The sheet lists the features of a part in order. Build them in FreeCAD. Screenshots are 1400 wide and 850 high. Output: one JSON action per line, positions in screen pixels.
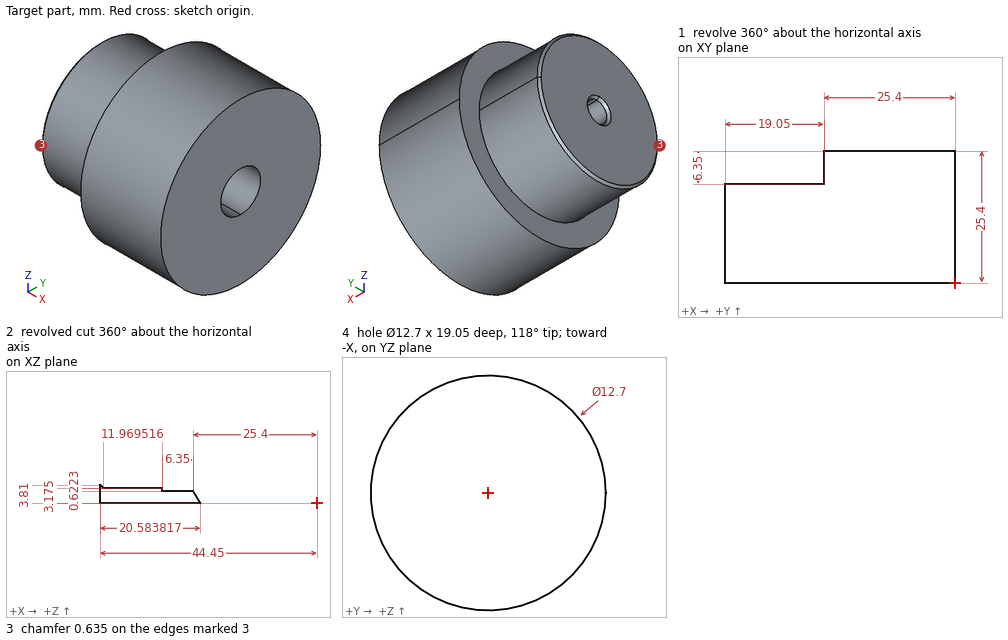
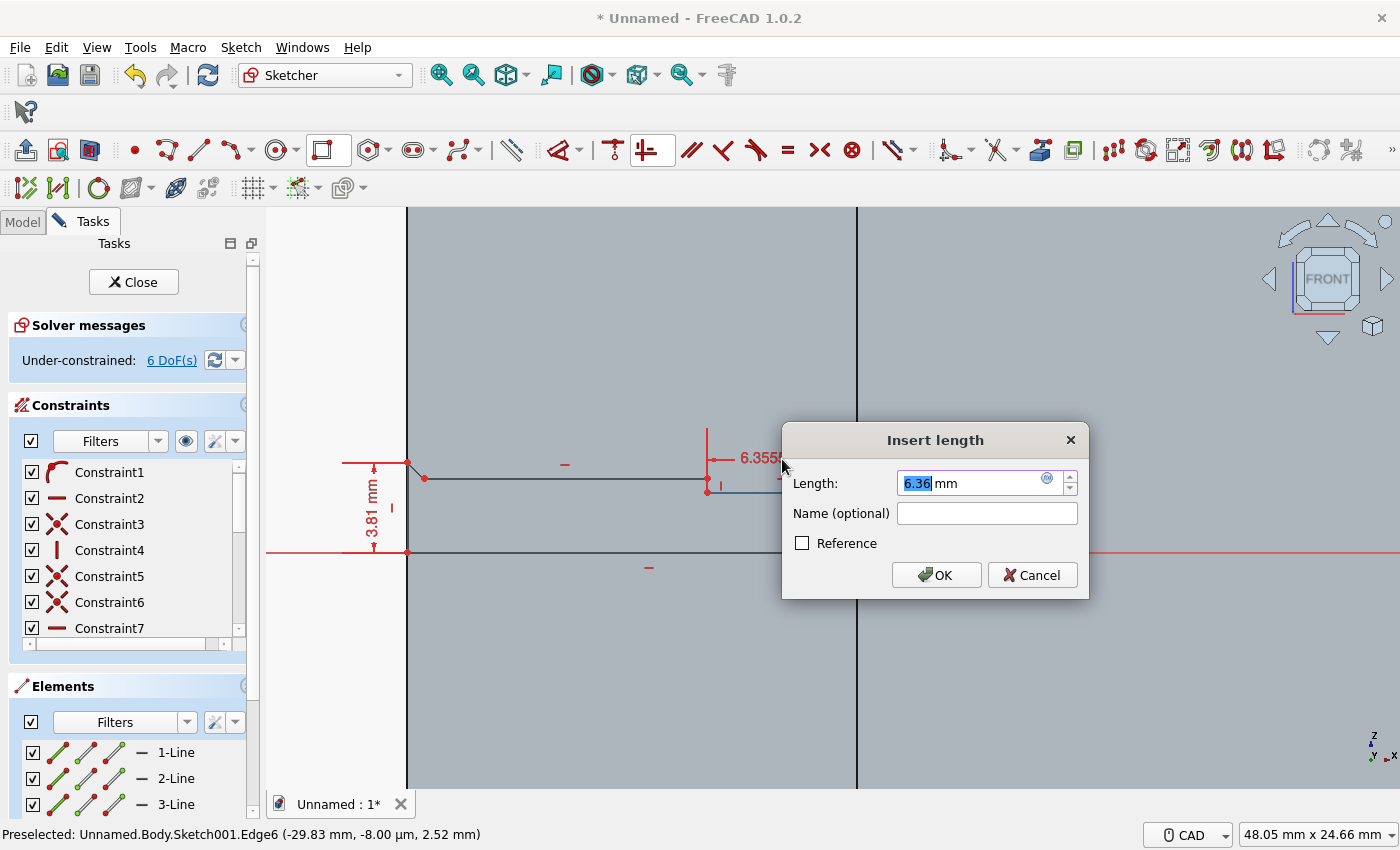
{"action": "type", "text": "6.35"}
{"action": "key", "text": "Return"}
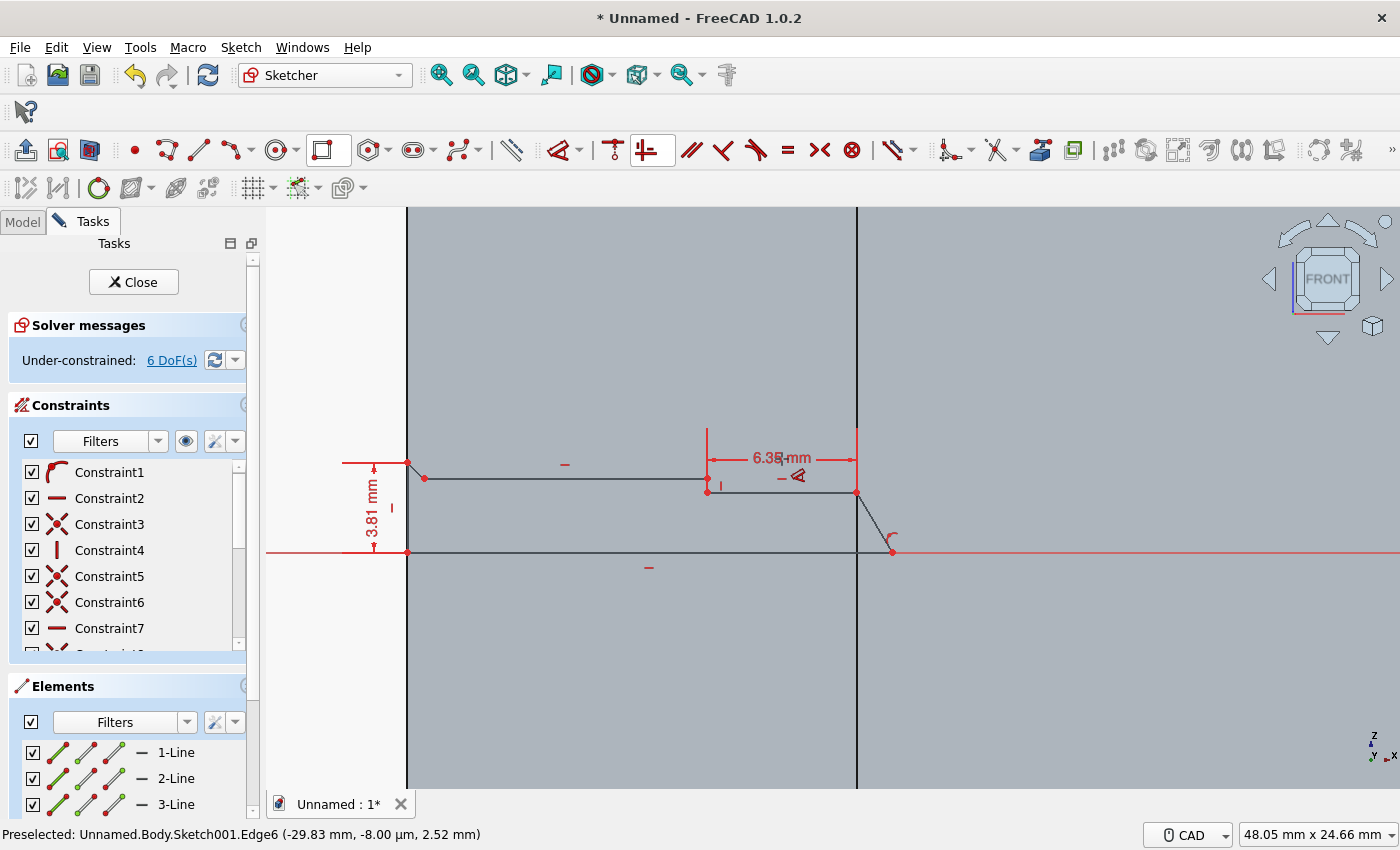
{"action": "left_click", "coordinate": [857, 493]}
{"action": "left_click", "coordinate": [1046, 587]}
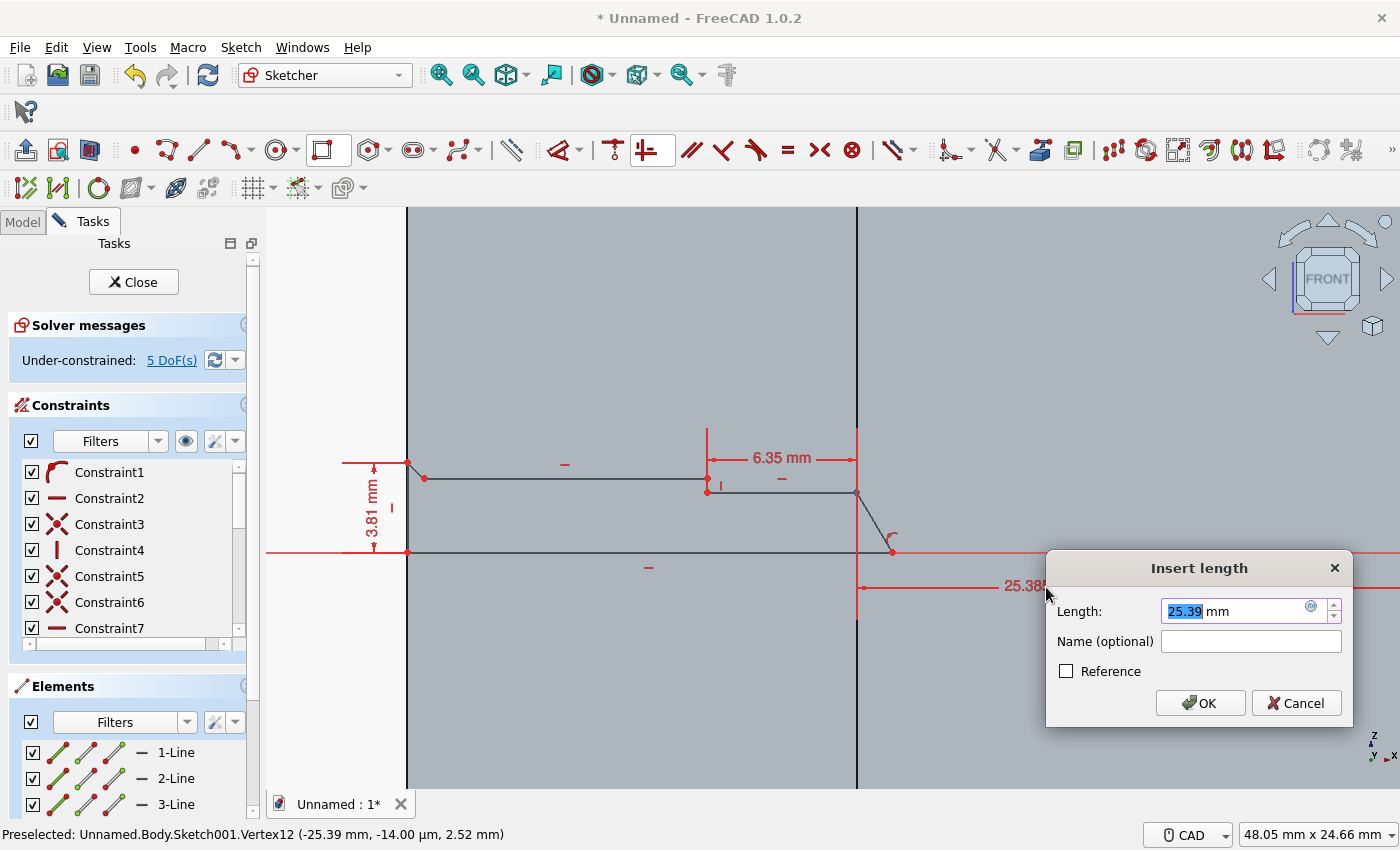
{"action": "type", "text": "25.4"}
{"action": "key", "text": "Return"}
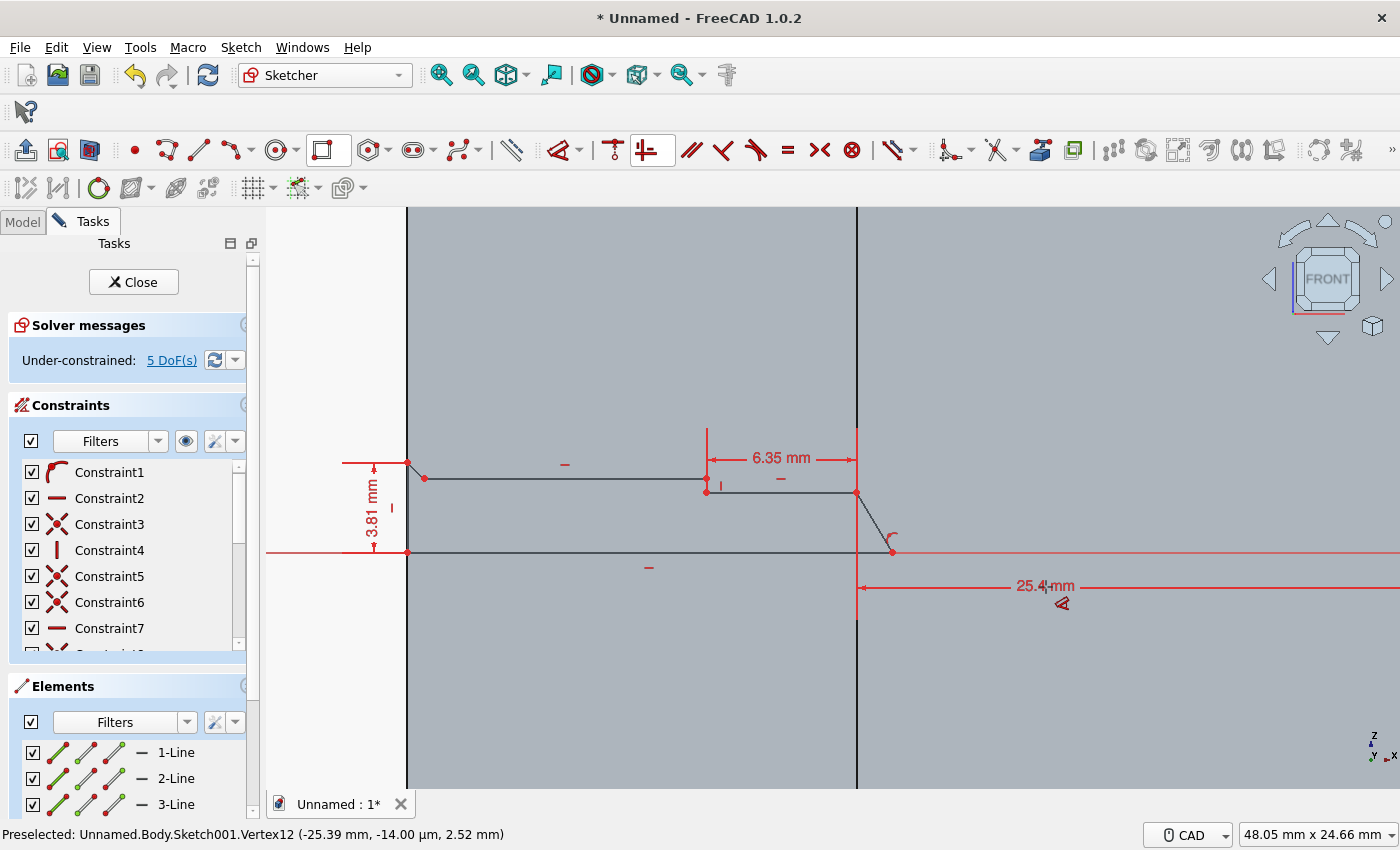
{"action": "scroll", "coordinate": [707, 486], "scroll_direction": "up", "scroll_amount": 5}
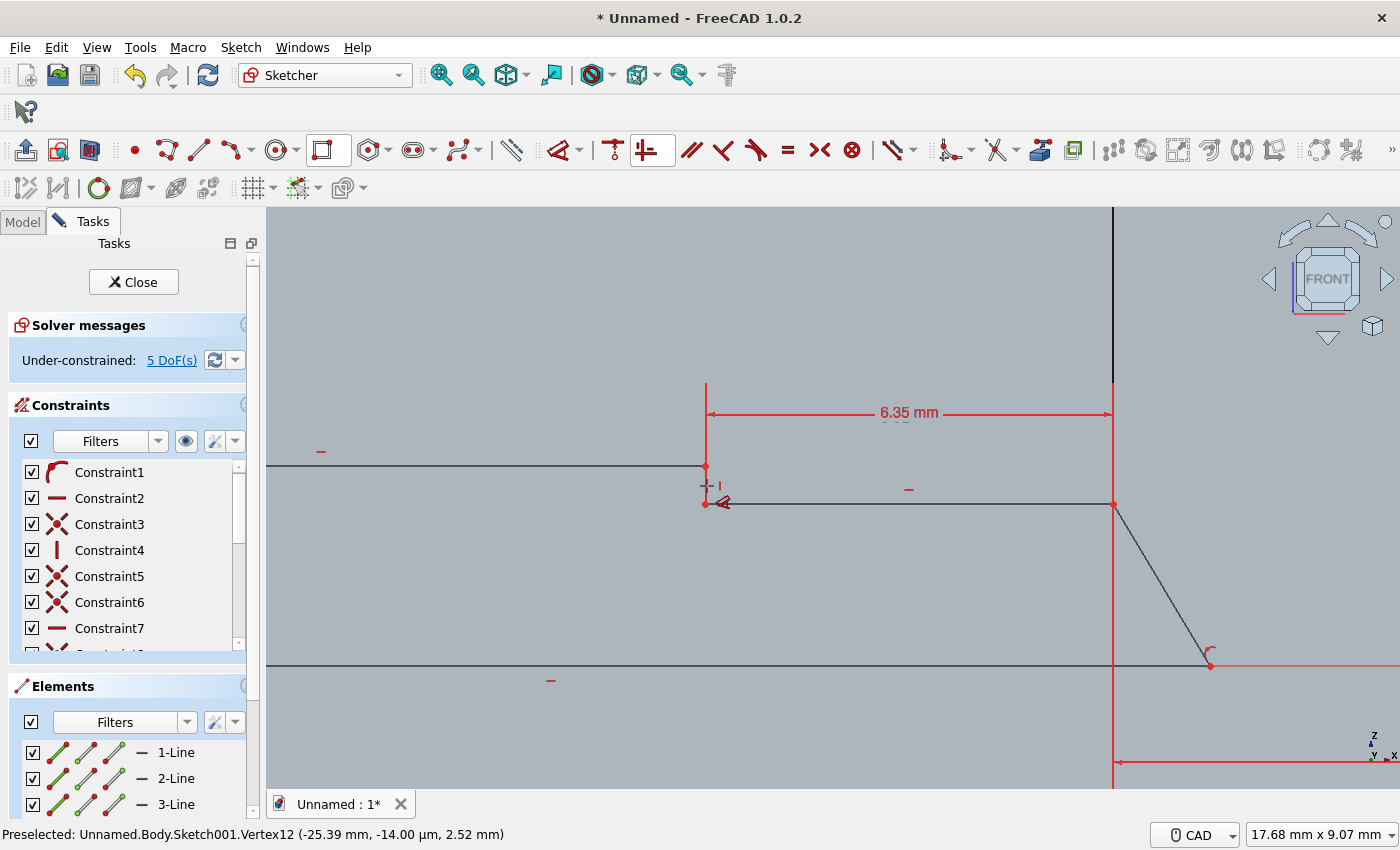
{"action": "left_click", "coordinate": [706, 485]}
{"action": "left_click", "coordinate": [672, 485]}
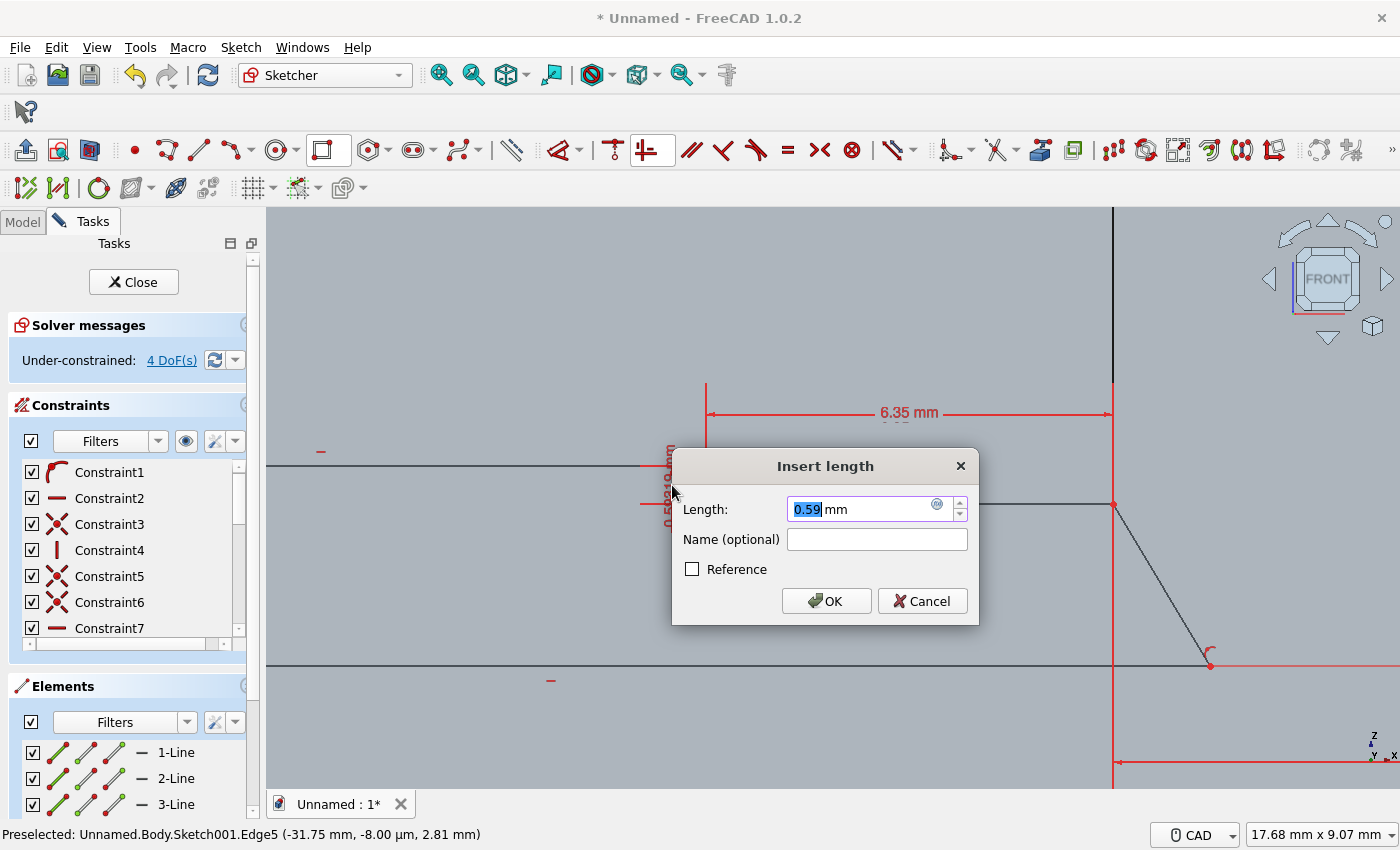
{"action": "type", "text": "0.6223"}
{"action": "key", "text": "Return"}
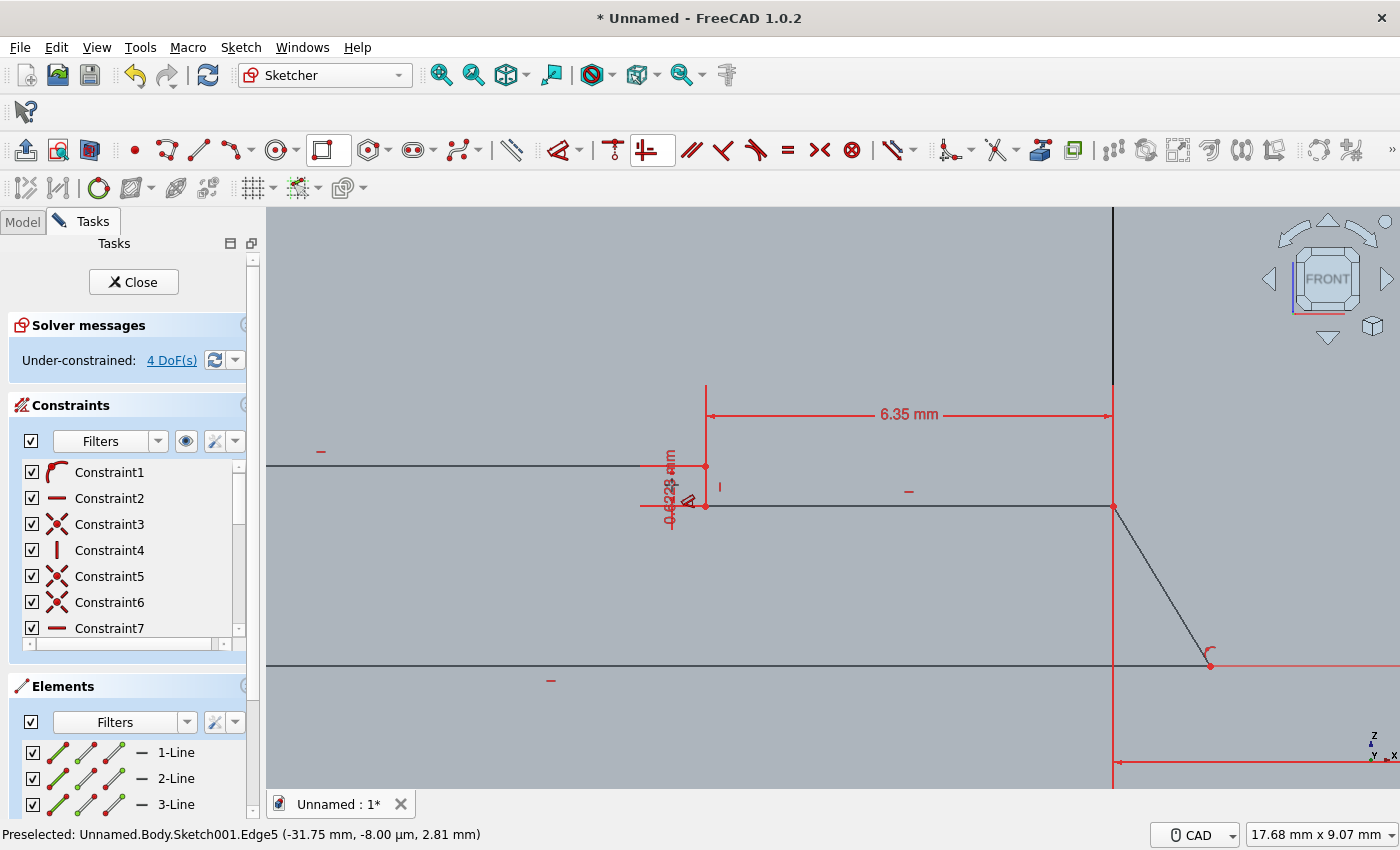
{"action": "scroll", "coordinate": [584, 483], "scroll_direction": "down", "scroll_amount": 7}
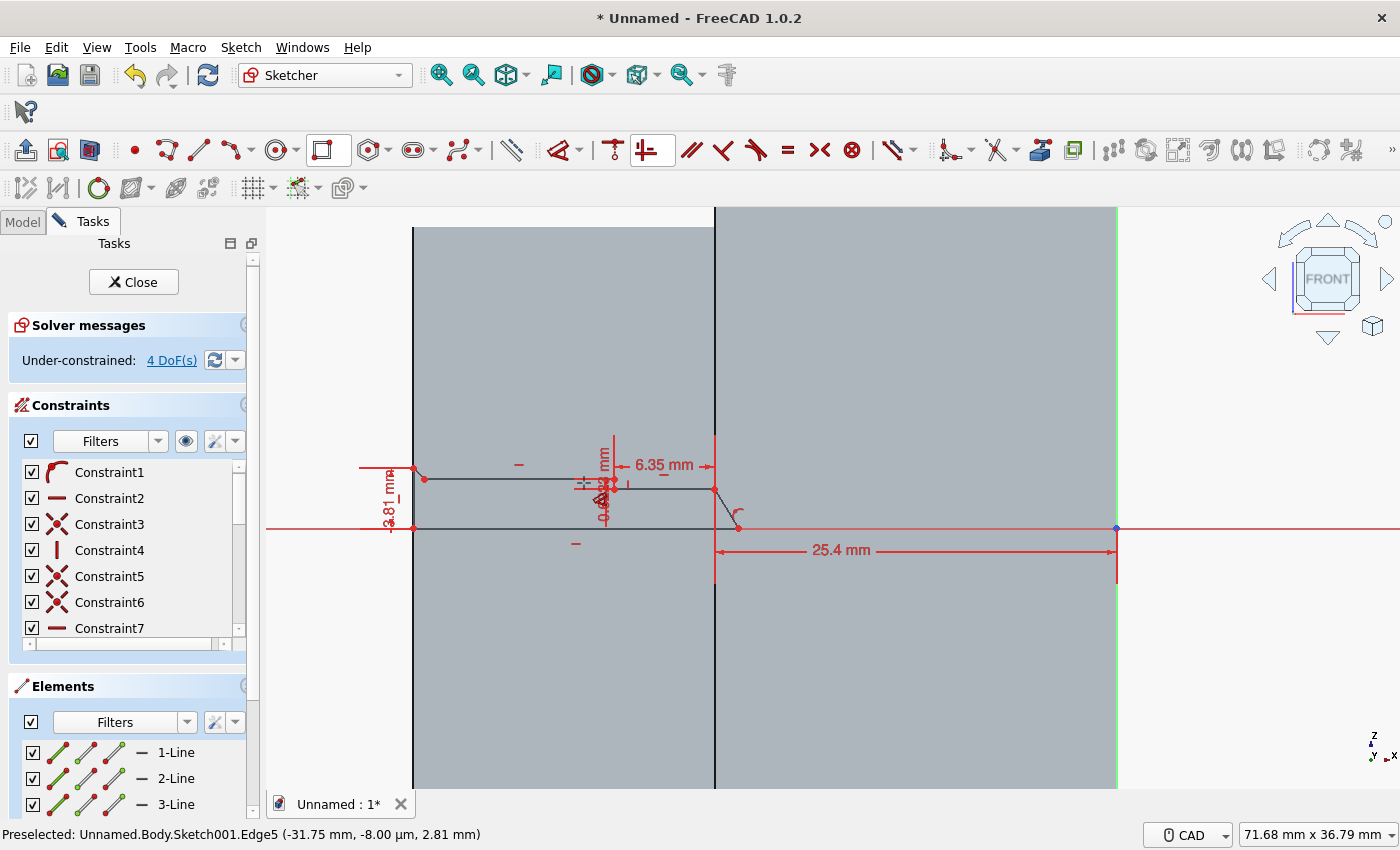
{"action": "left_click", "coordinate": [414, 528]}
{"action": "left_click", "coordinate": [765, 562]}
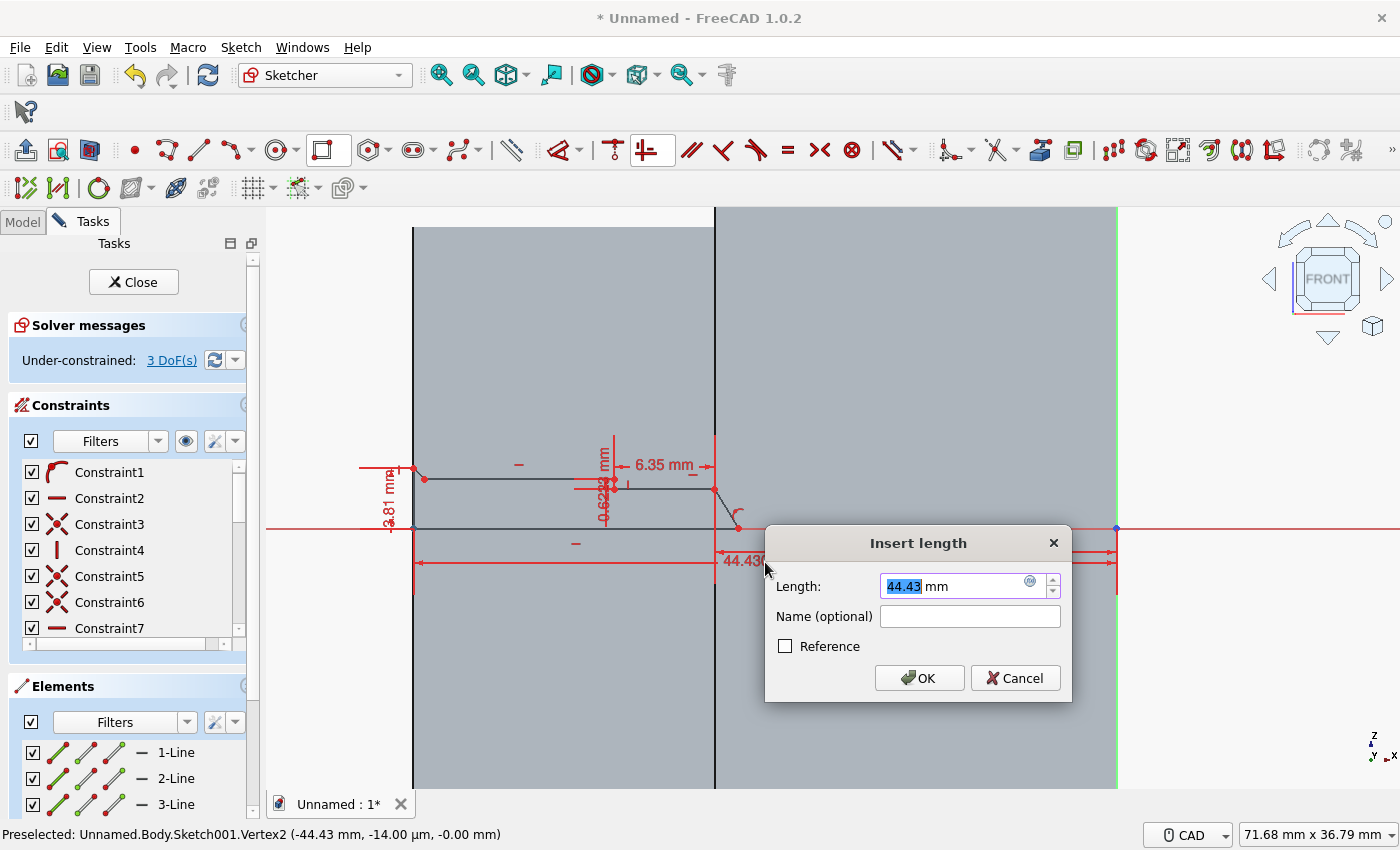
{"action": "type", "text": "44.45"}
{"action": "key", "text": "Return"}